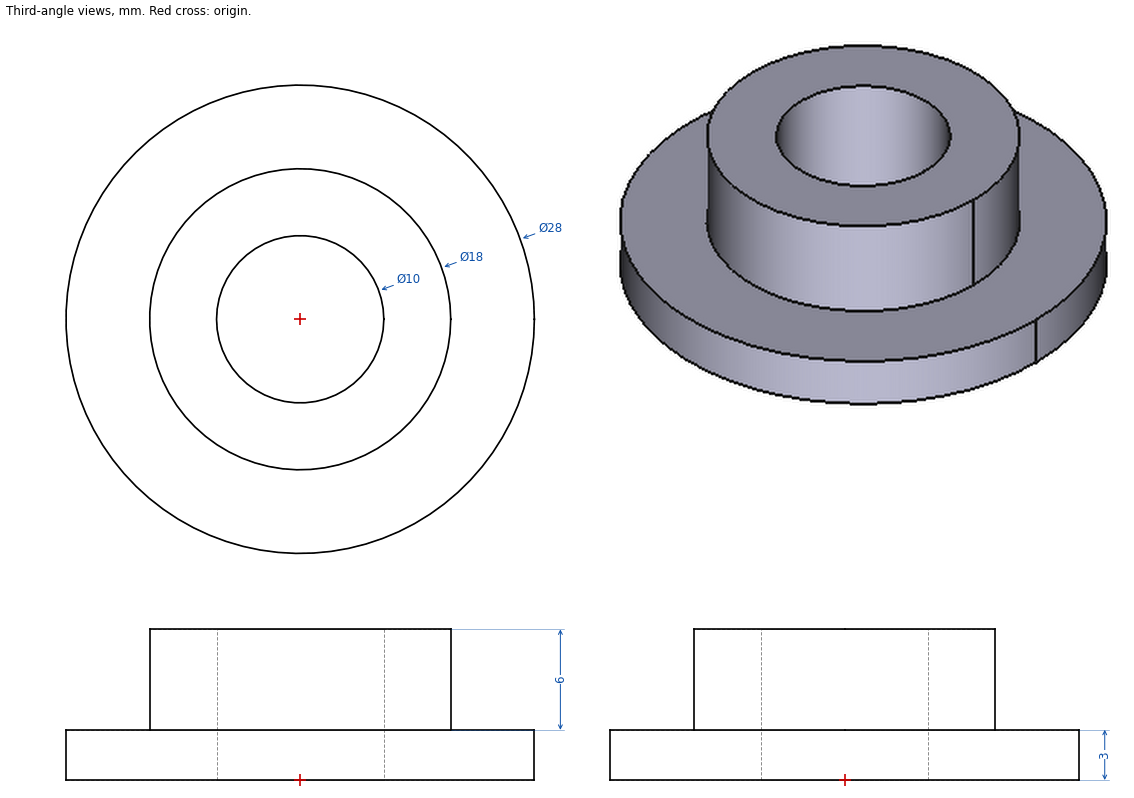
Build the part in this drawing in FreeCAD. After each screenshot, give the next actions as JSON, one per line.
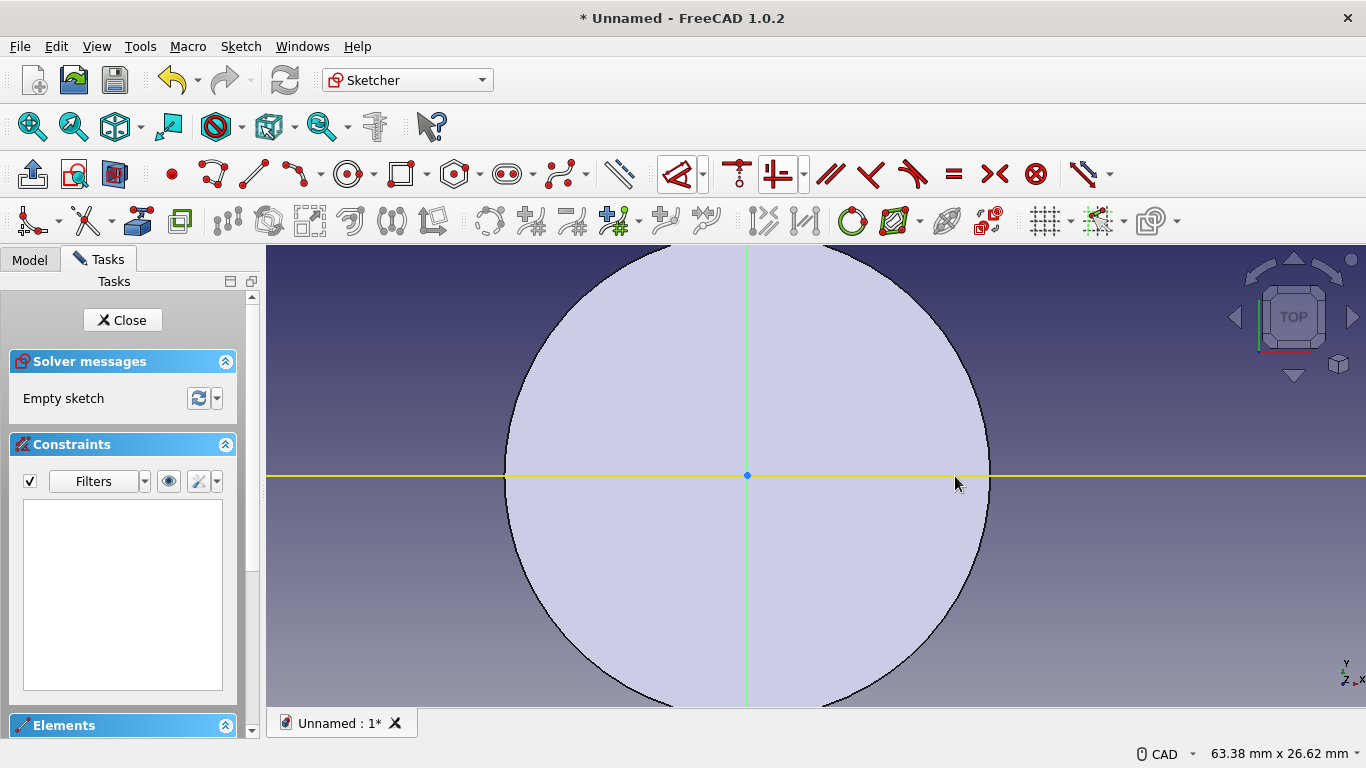
{"action": "key", "text": "g c"}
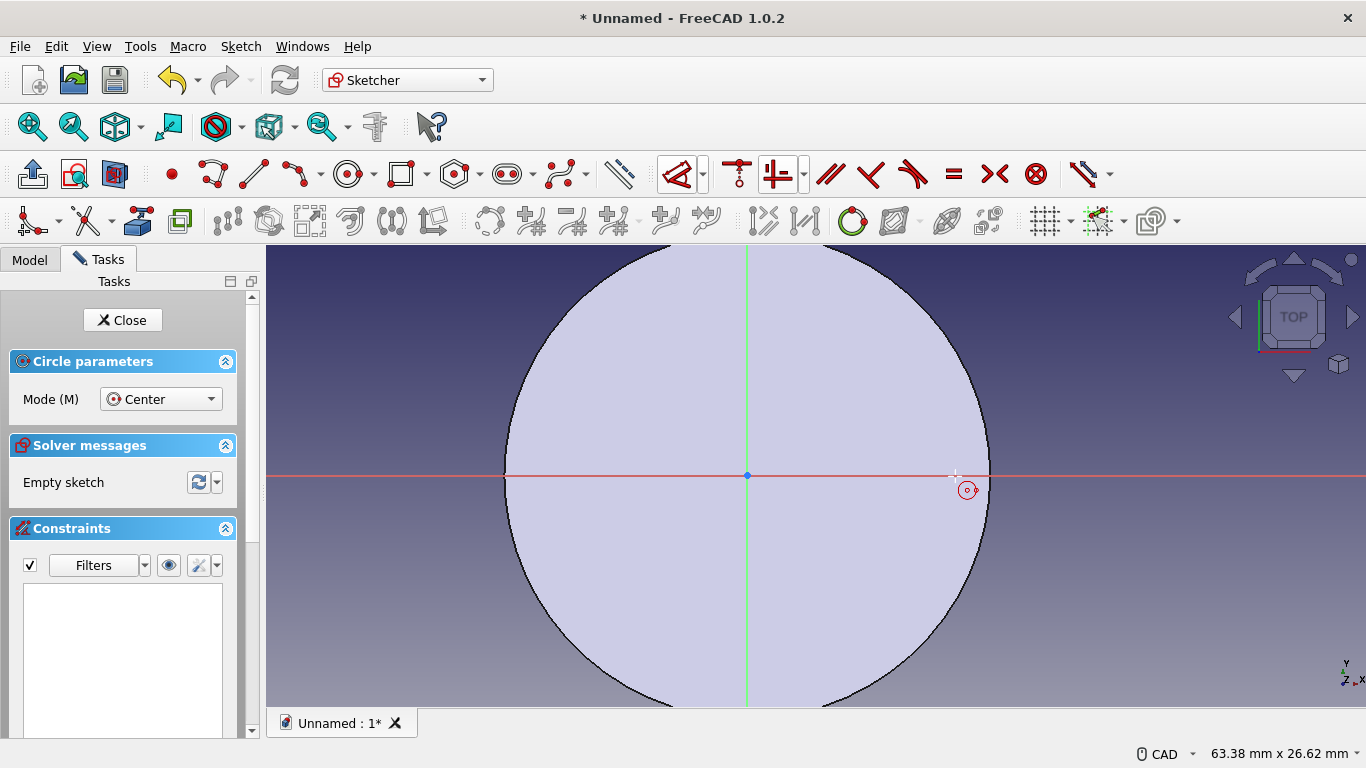
{"action": "left_click", "coordinate": [747, 476]}
{"action": "left_click", "coordinate": [858, 365]}
{"action": "key", "text": "Escape"}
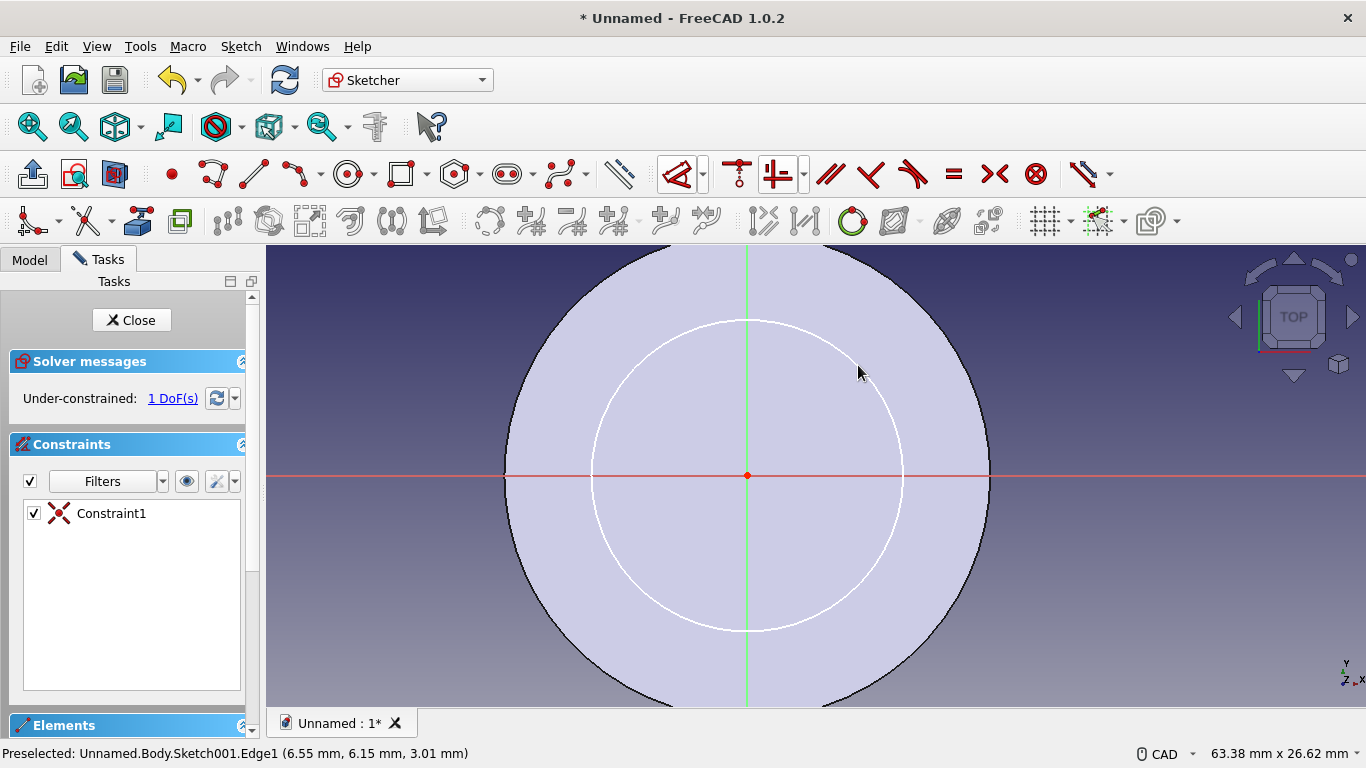
{"action": "left_click", "coordinate": [857, 365]}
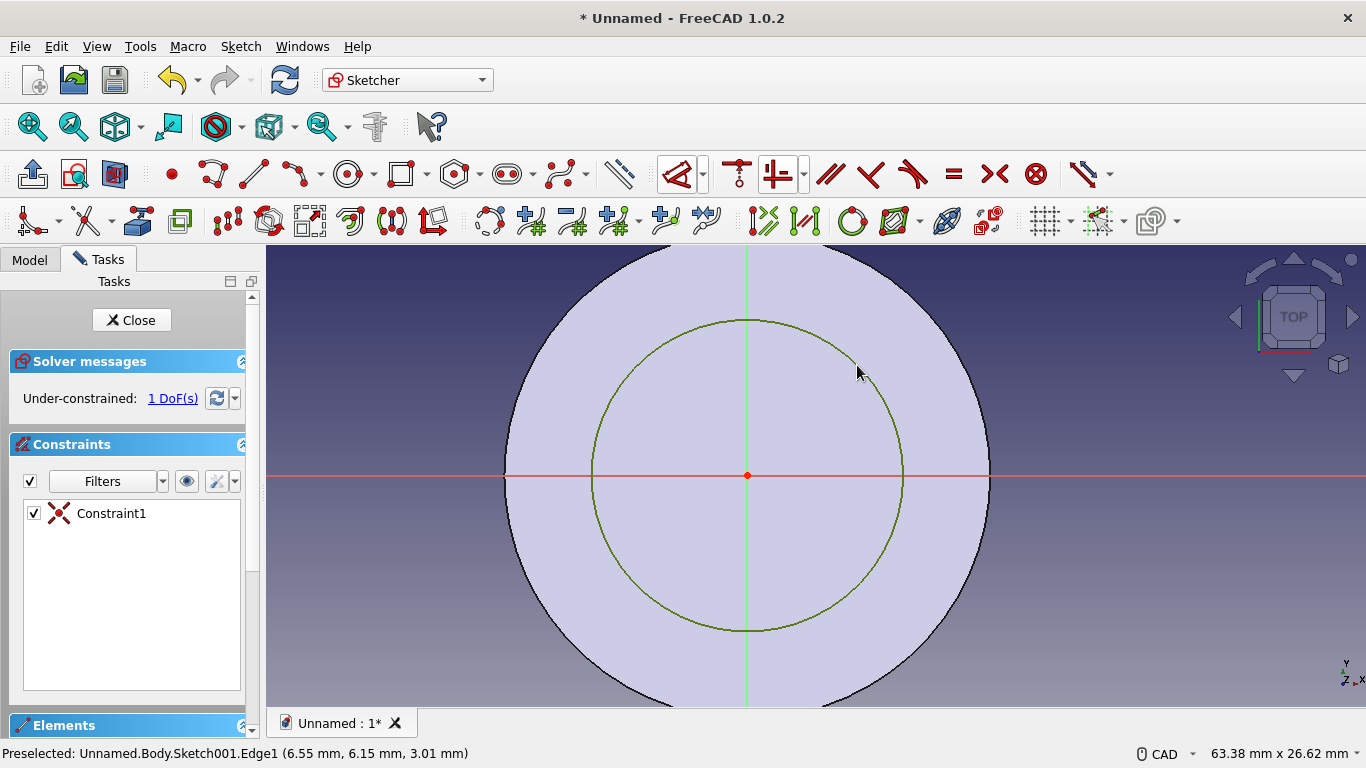
{"action": "key", "text": "k o"}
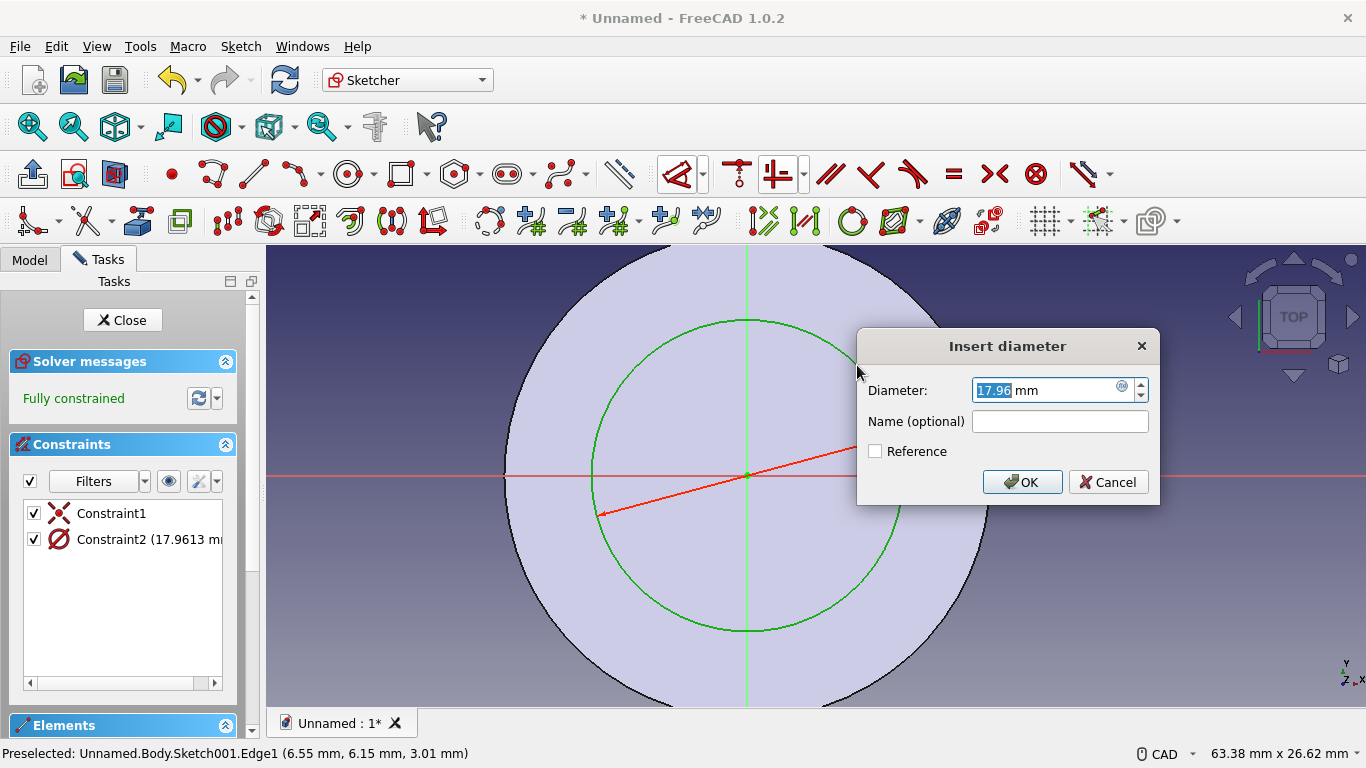
{"action": "type", "text": "18"}
{"action": "key", "text": "Return"}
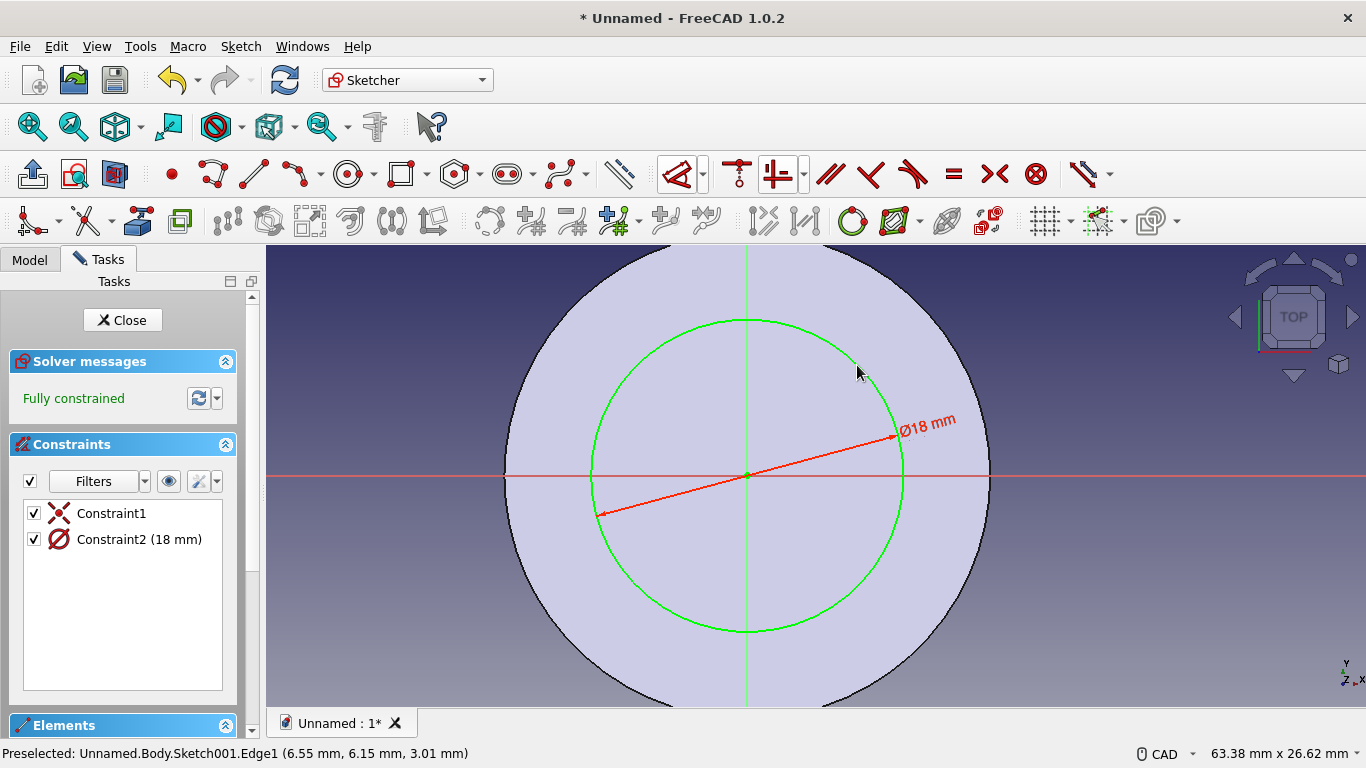
{"action": "left_click", "coordinate": [123, 320]}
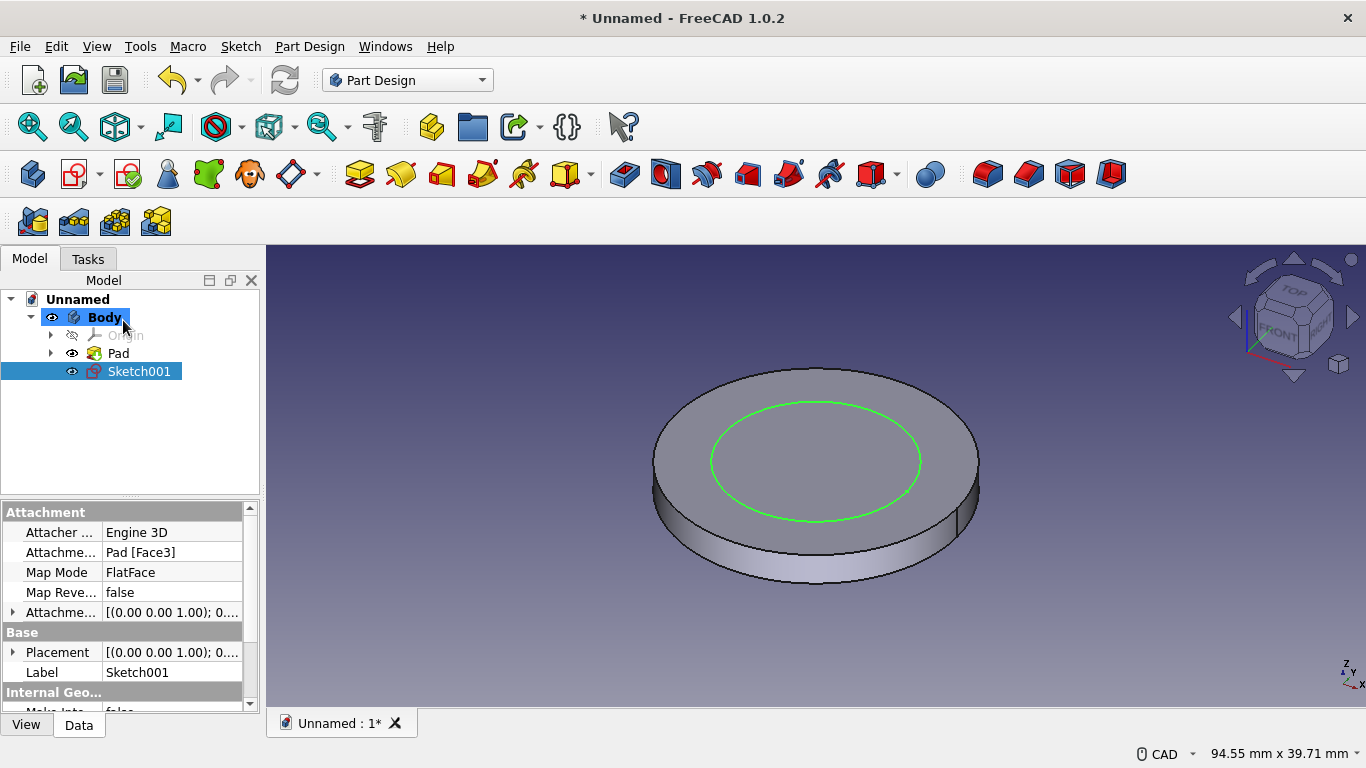
{"action": "left_click", "coordinate": [360, 174]}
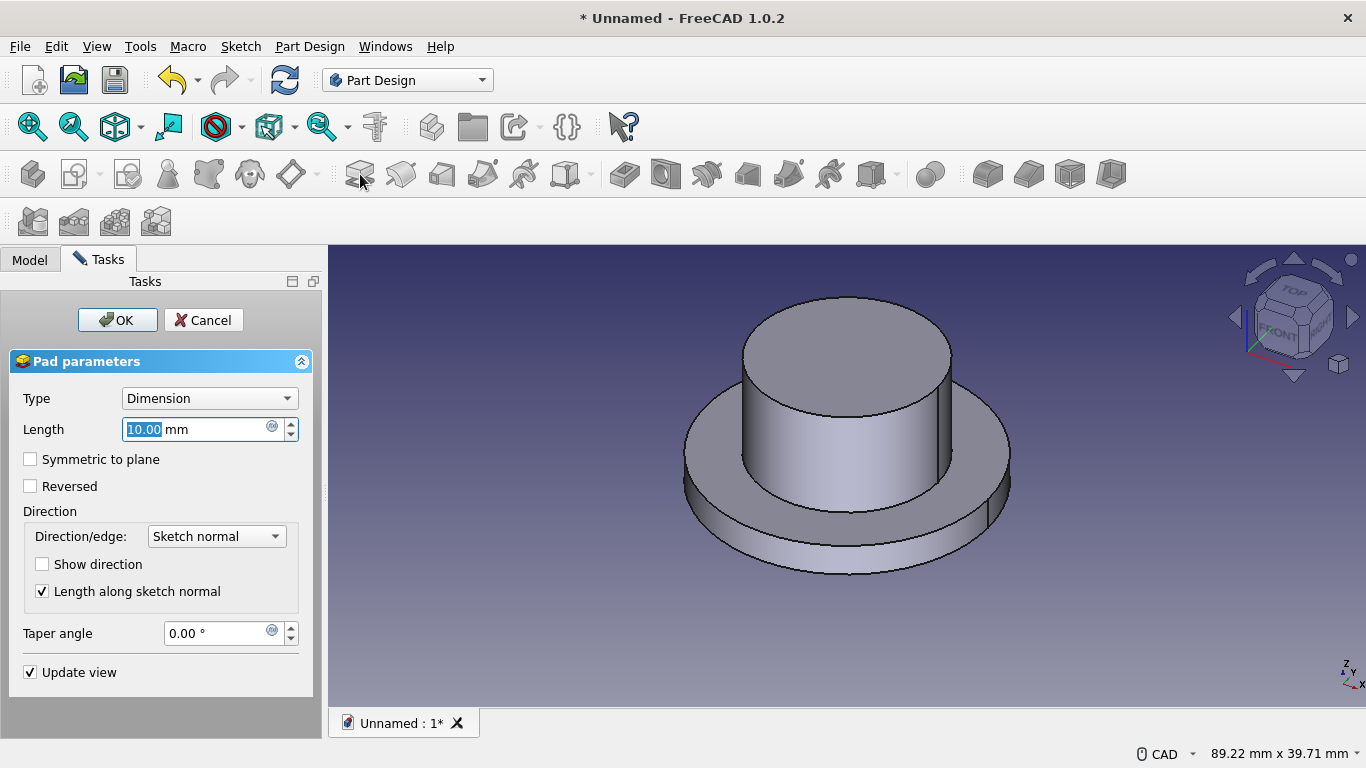
{"action": "type", "text": "6"}
{"action": "key", "text": "Tab"}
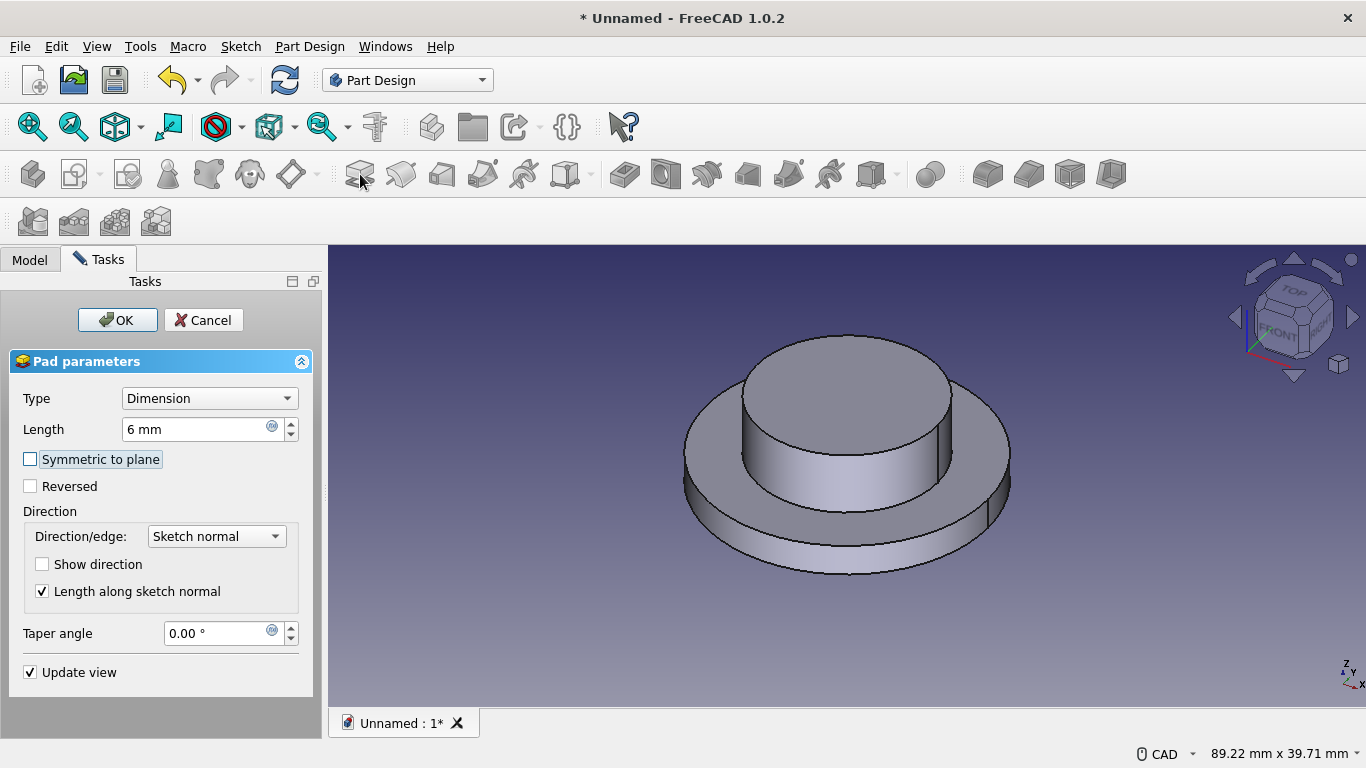
{"action": "left_click", "coordinate": [118, 320]}